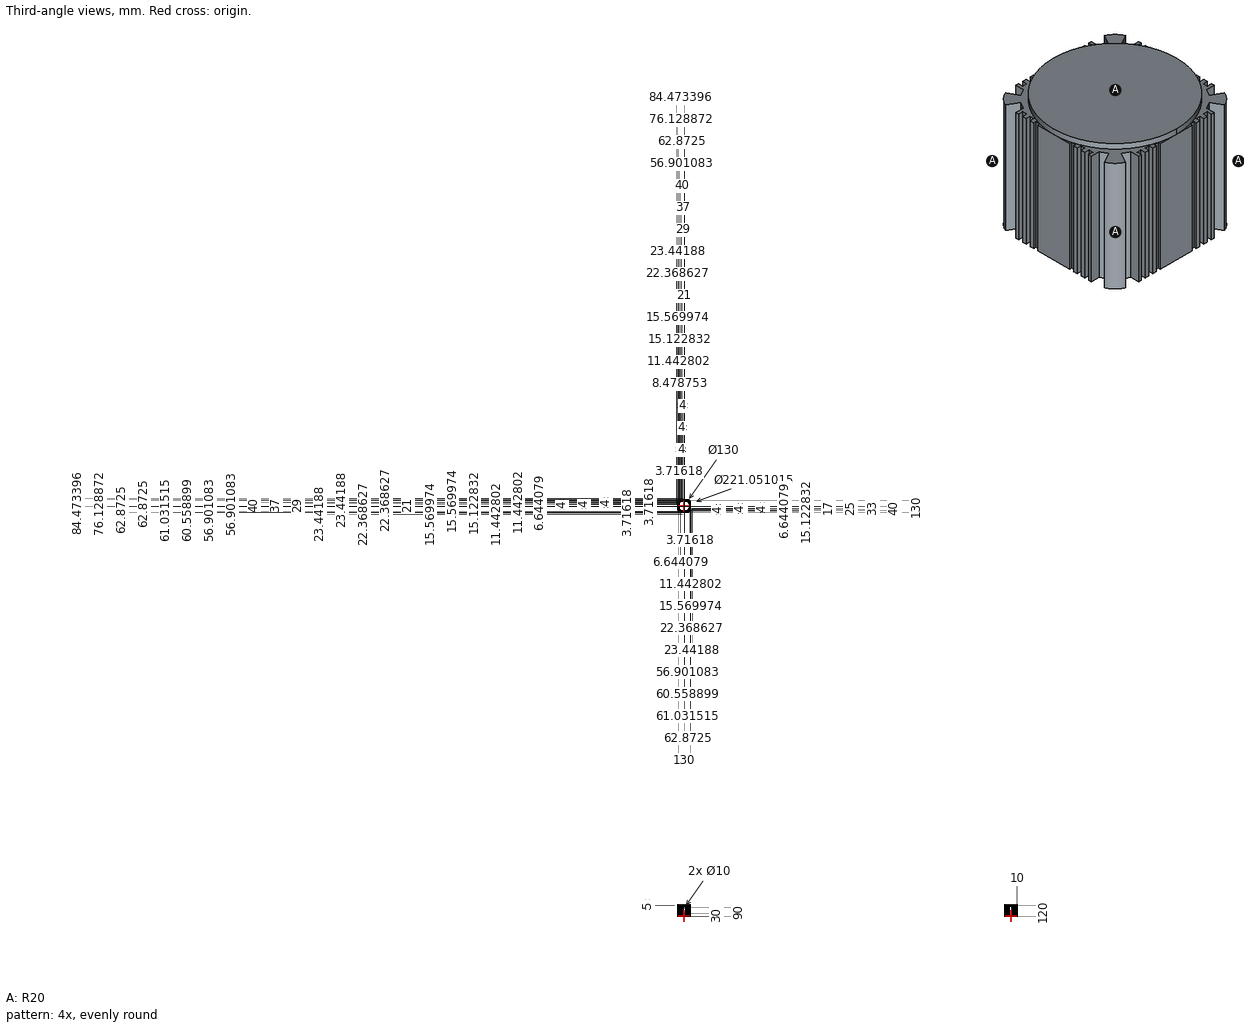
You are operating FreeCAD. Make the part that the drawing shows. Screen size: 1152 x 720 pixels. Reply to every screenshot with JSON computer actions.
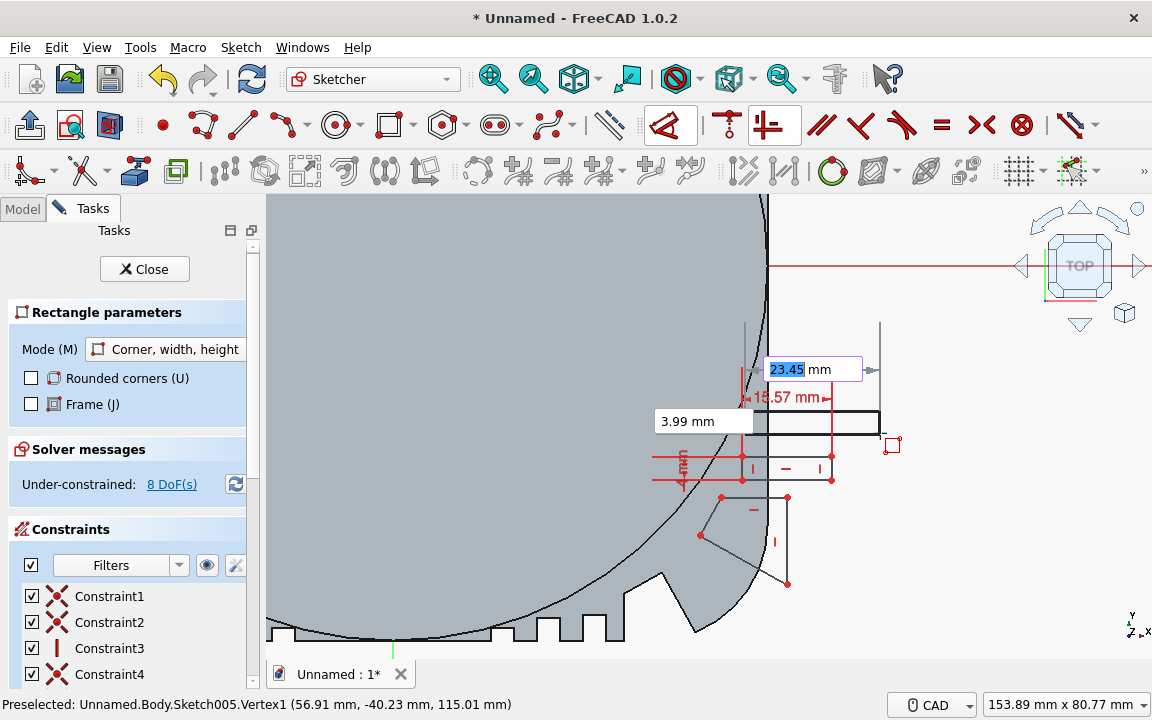
{"action": "type", "text": "23.44188"}
{"action": "key", "text": "Tab"}
{"action": "type", "text": "4"}
{"action": "key", "text": "Return"}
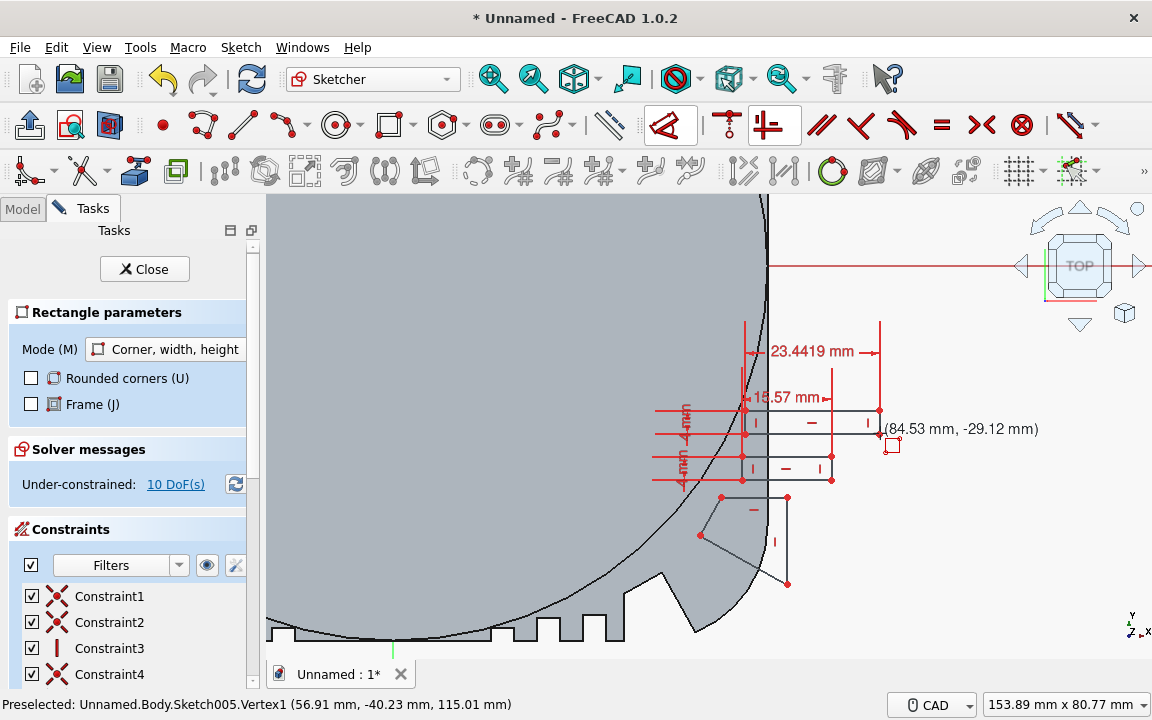
{"action": "left_click", "coordinate": [755, 364]}
{"action": "mouse_move", "coordinate": [884, 387]}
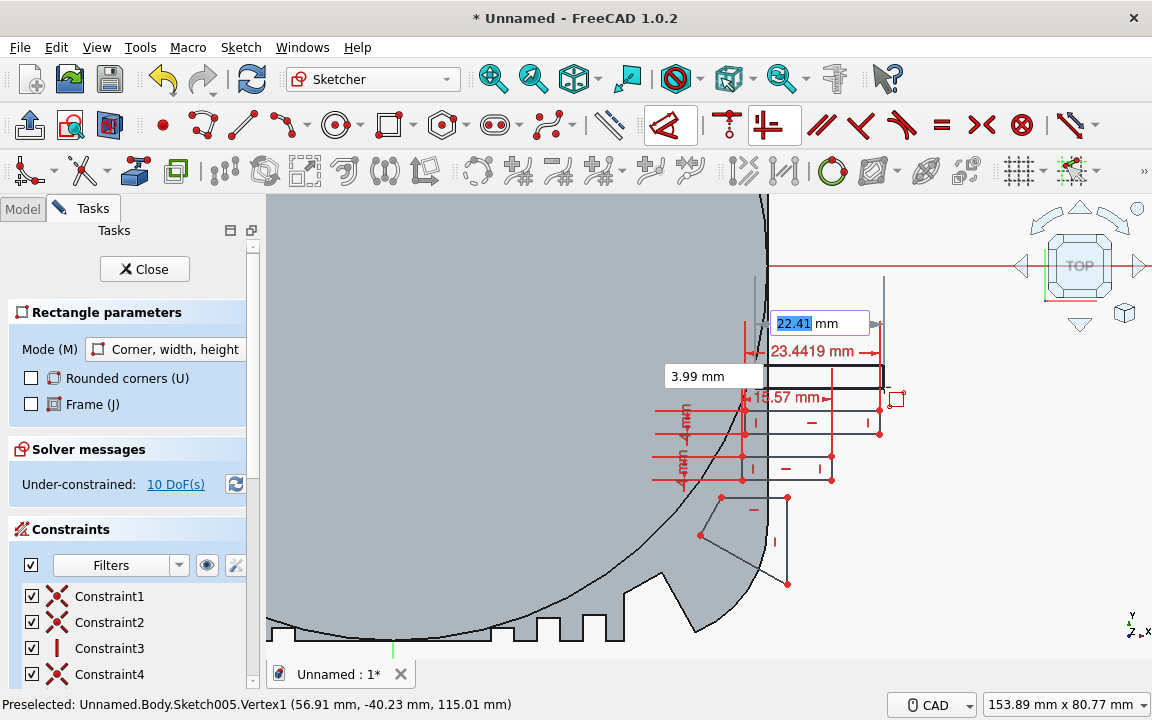
{"action": "type", "text": "22.368627"}
{"action": "key", "text": "Tab"}
{"action": "type", "text": "4"}
{"action": "key", "text": "Return"}
{"action": "key", "text": "Escape"}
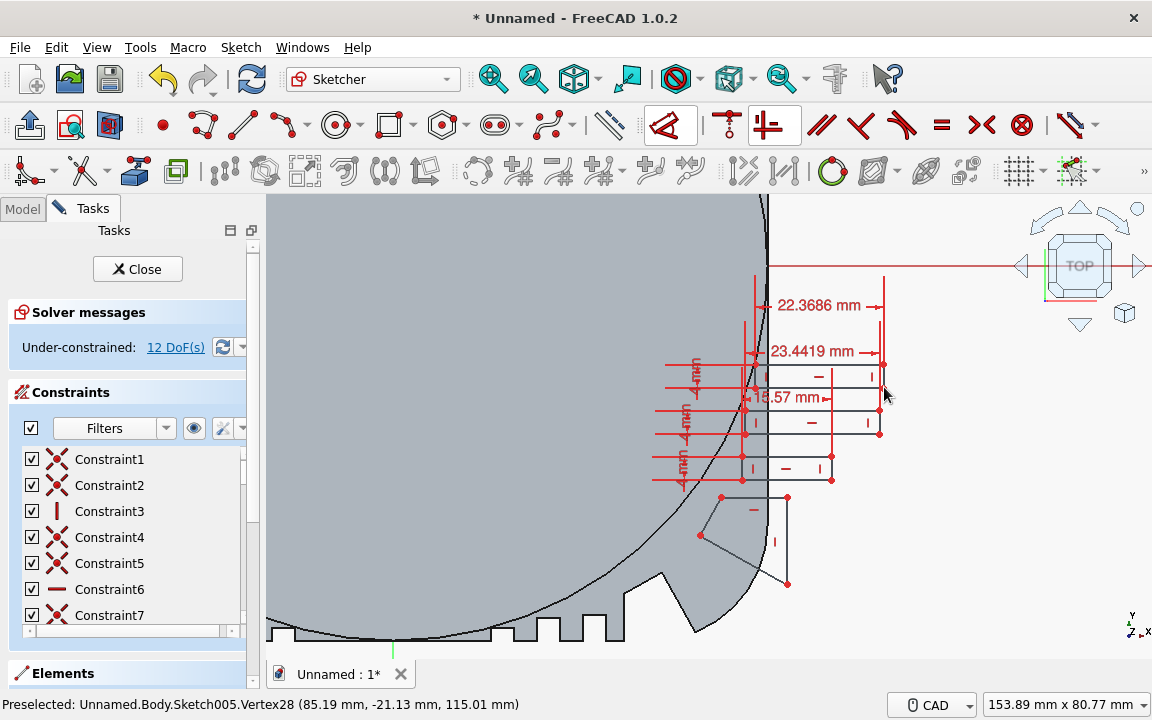
{"action": "left_click", "coordinate": [721, 498]}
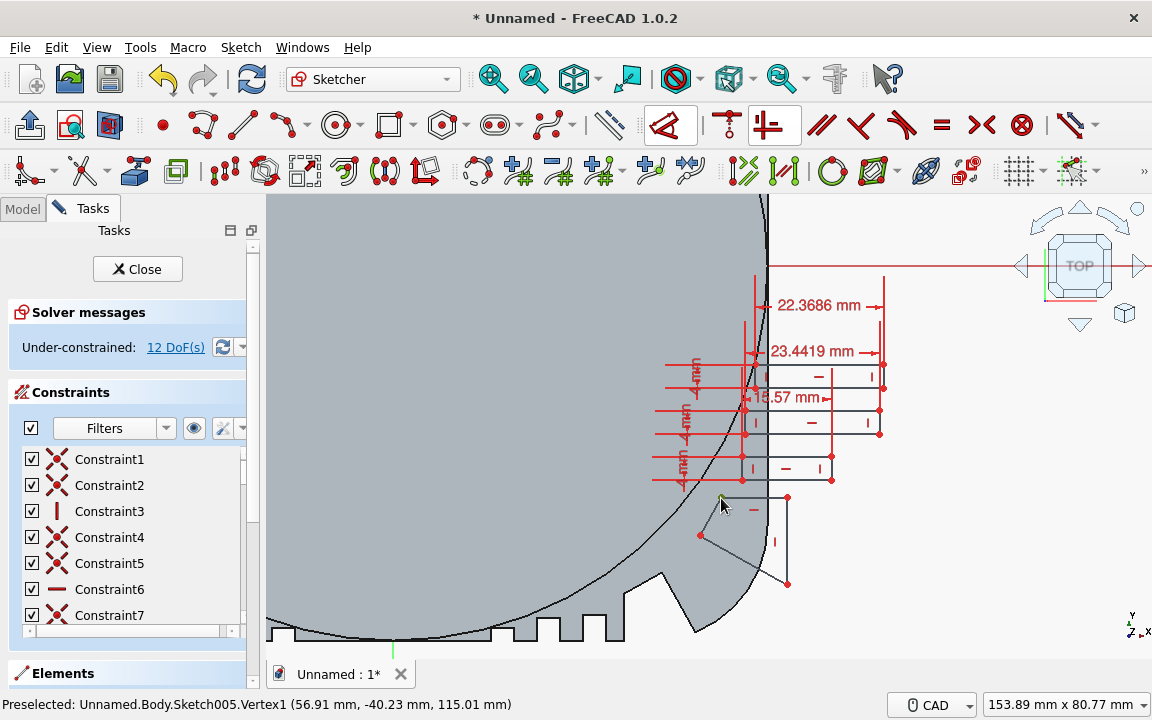
{"action": "key", "text": "i"}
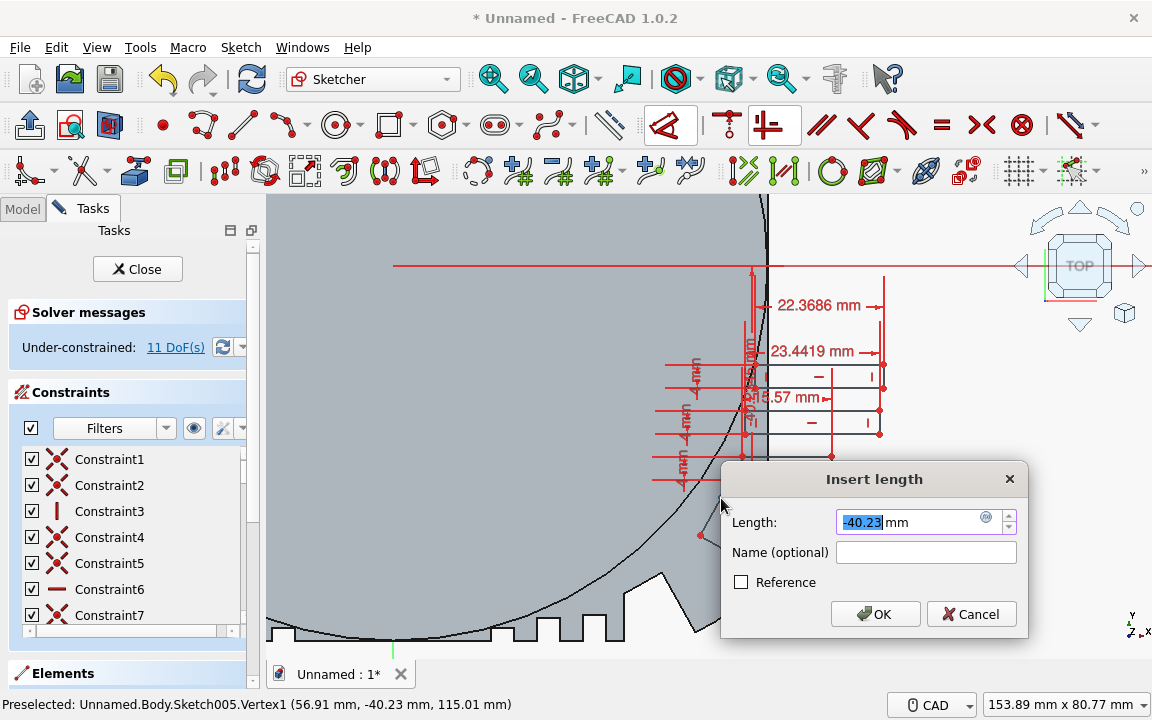
{"action": "type", "text": "-40"}
{"action": "key", "text": "Return"}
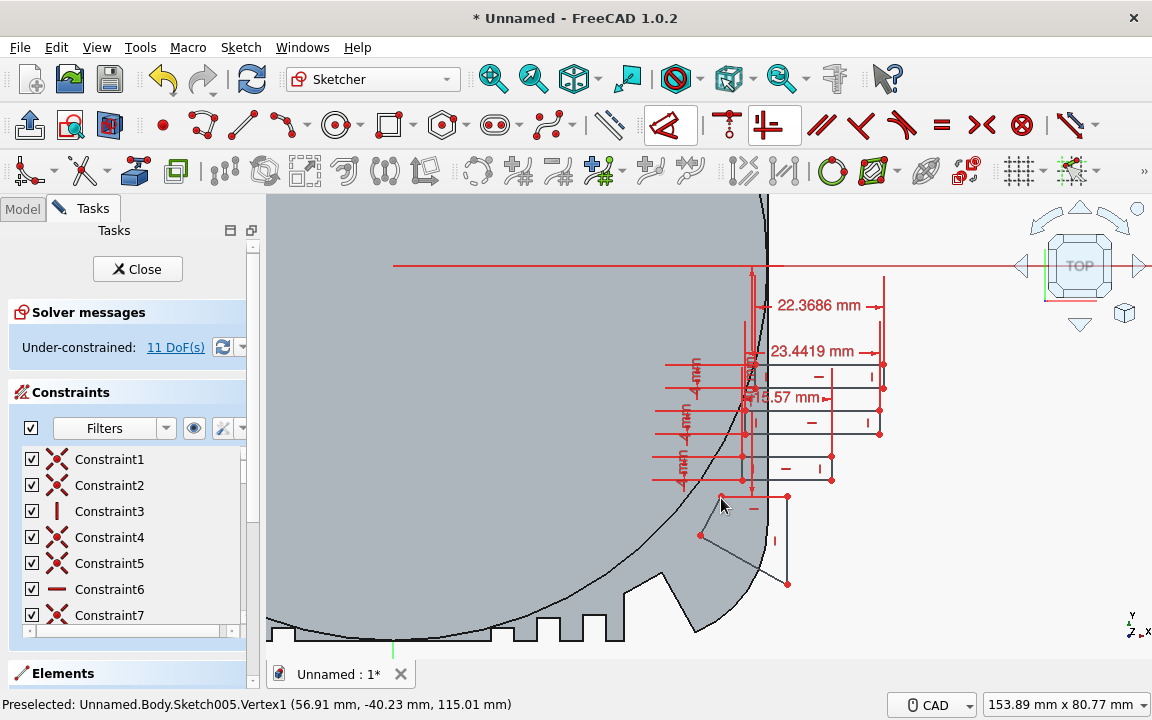
{"action": "left_click", "coordinate": [742, 457]}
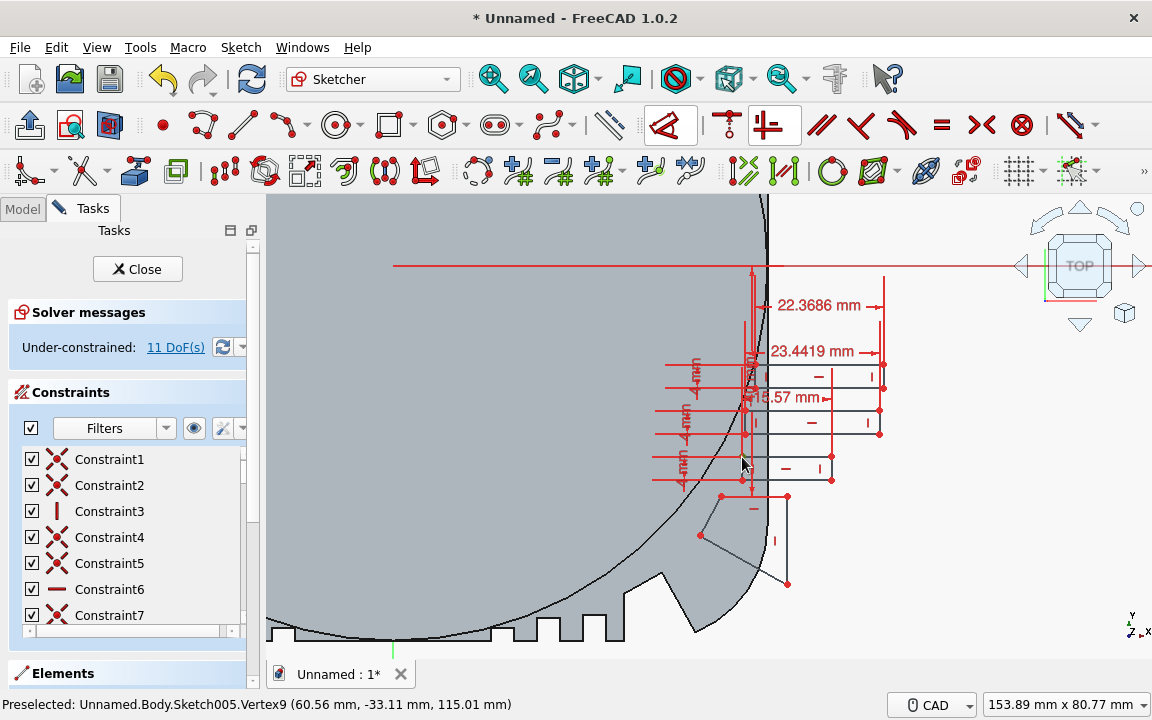
{"action": "left_click", "coordinate": [692, 126]}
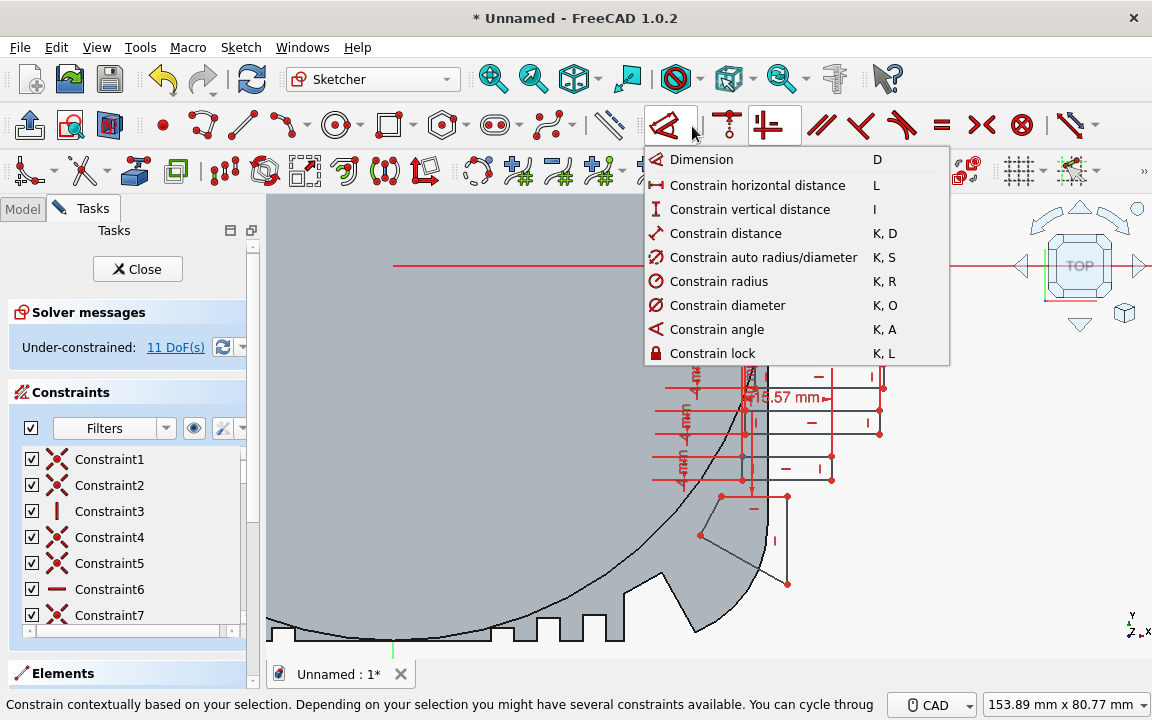
{"action": "left_click", "coordinate": [797, 209]}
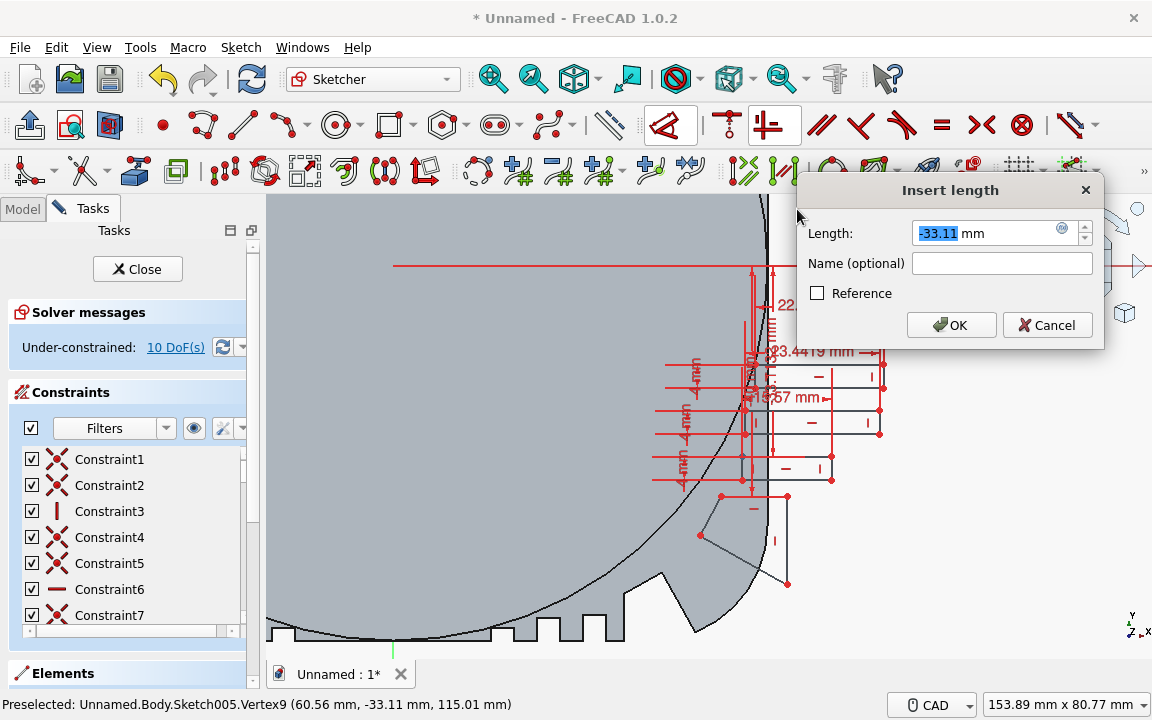
{"action": "type", "text": "-33"}
{"action": "key", "text": "Return"}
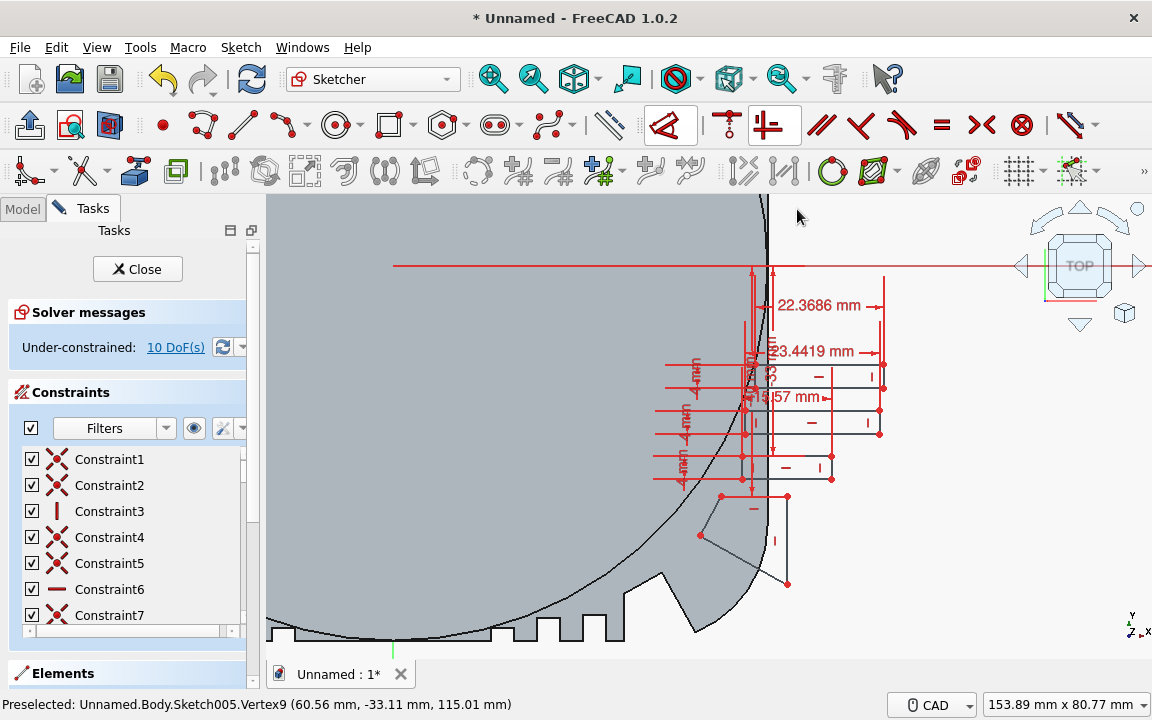
{"action": "left_click", "coordinate": [745, 411]}